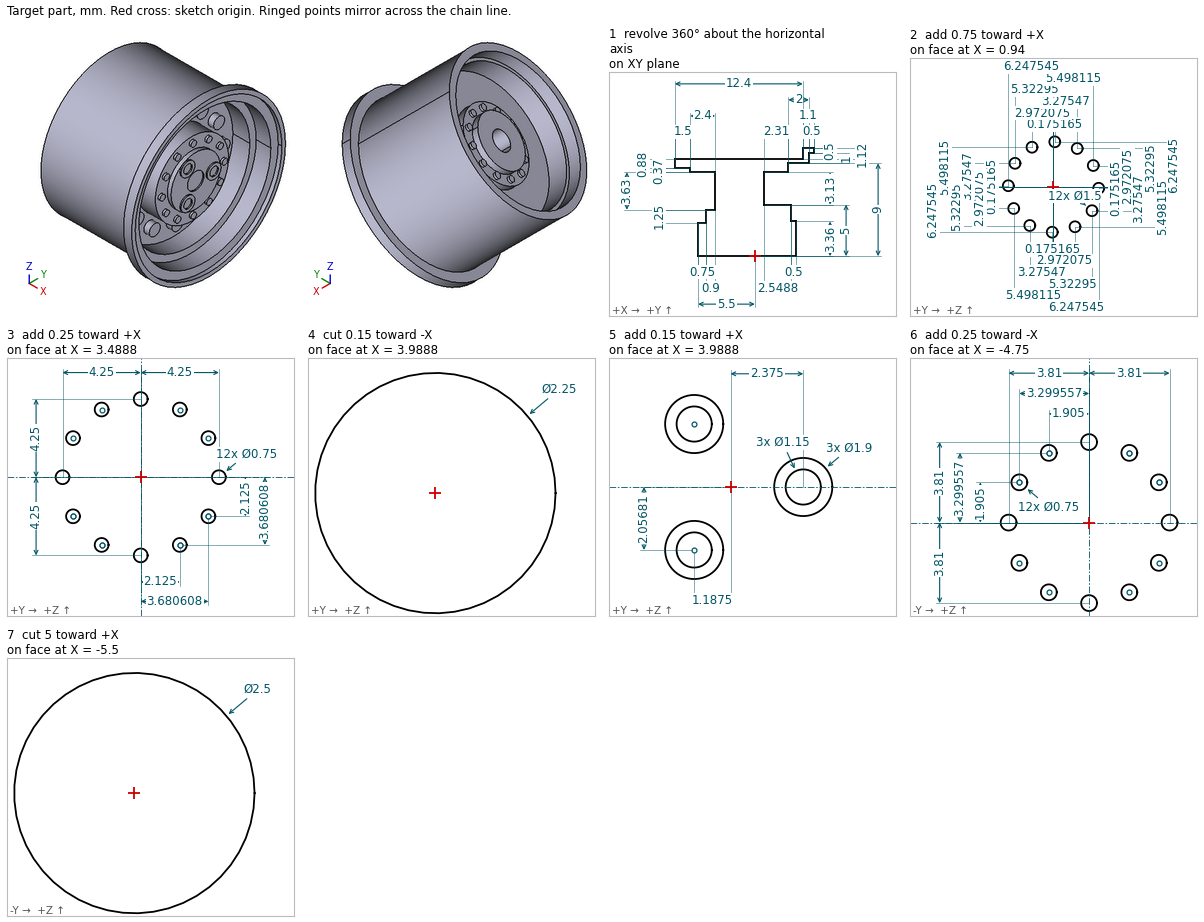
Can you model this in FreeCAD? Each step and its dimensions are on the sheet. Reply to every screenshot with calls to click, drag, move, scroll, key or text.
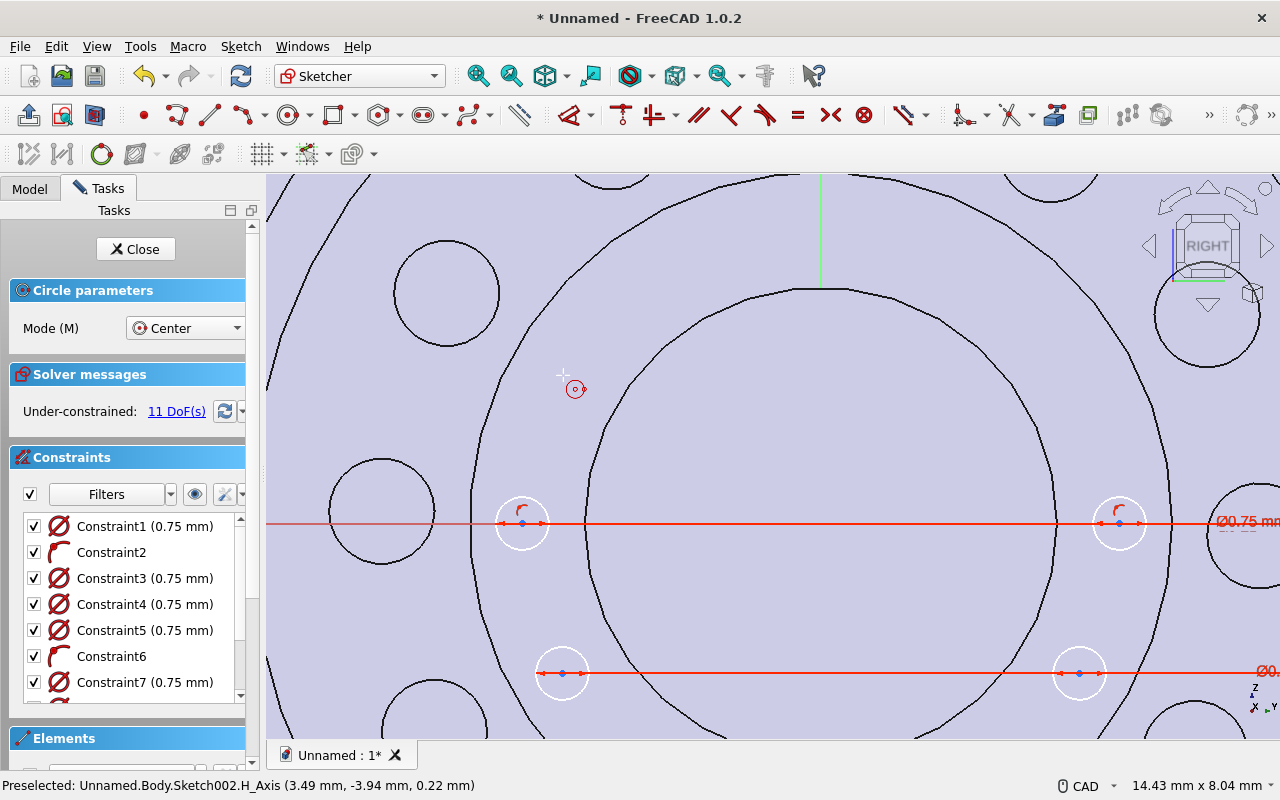
click(562, 374)
move(581, 356)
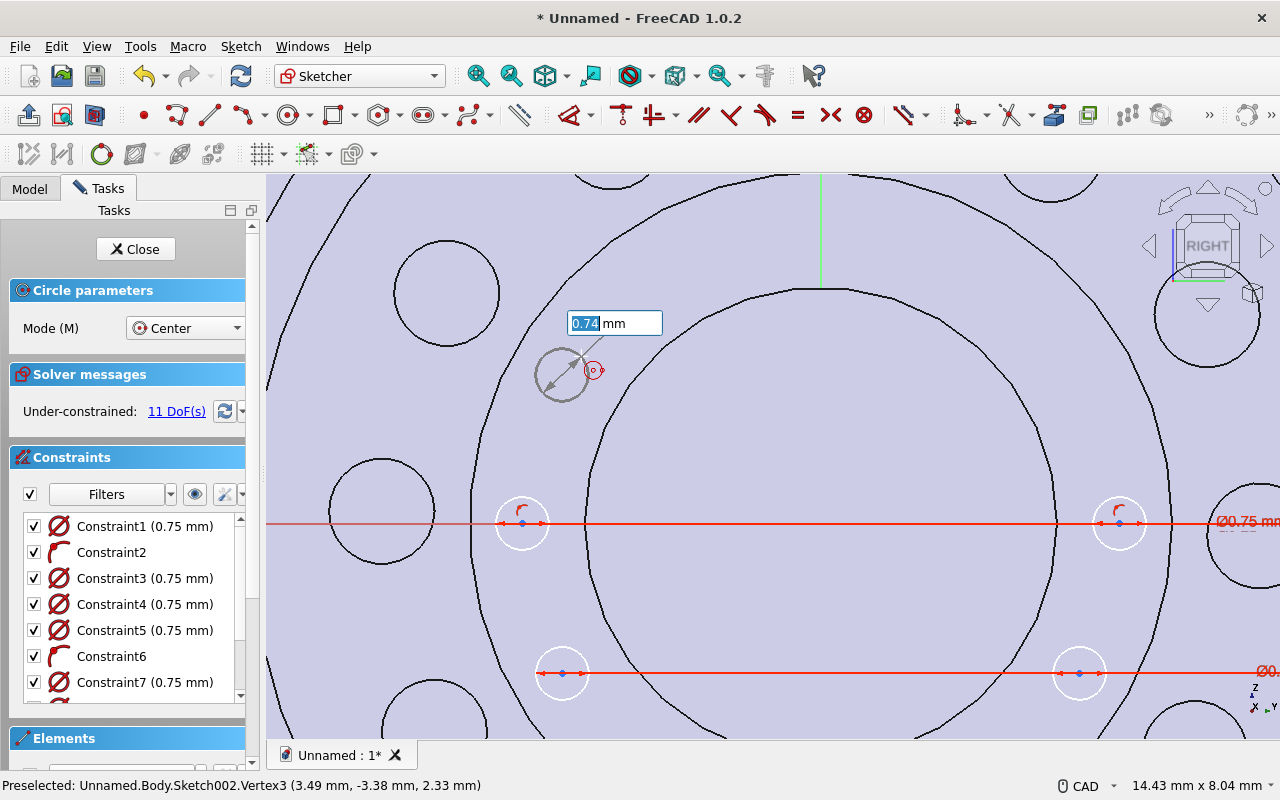
text(0.75)
key(Return)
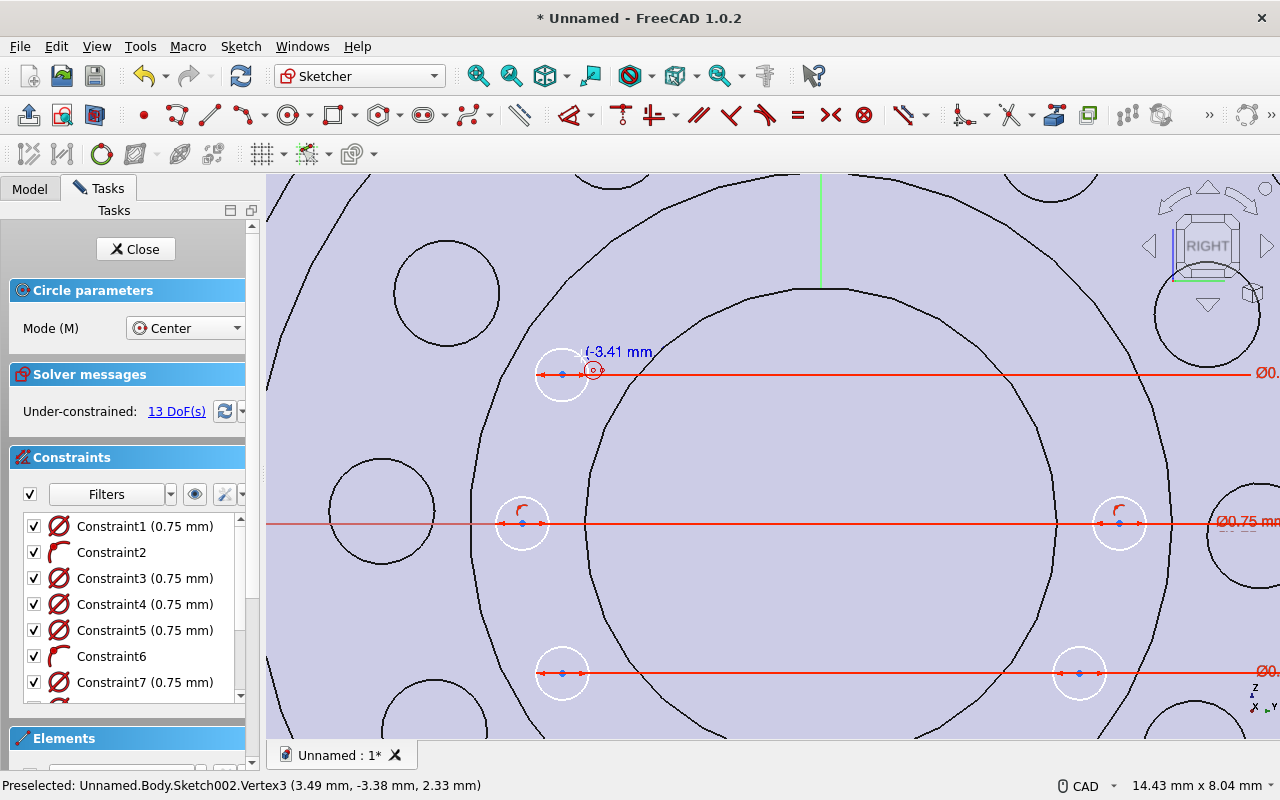
click(671, 265)
move(690, 246)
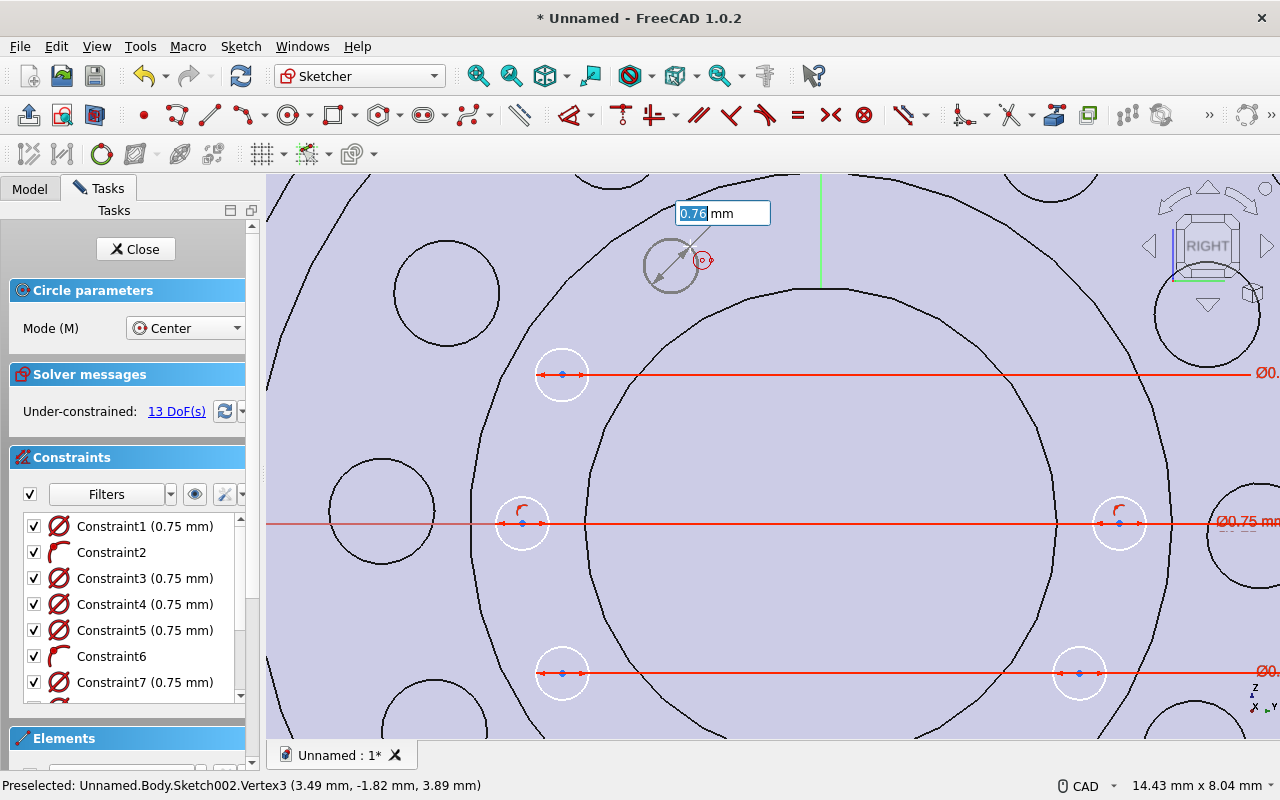
text(0.75)
key(Return)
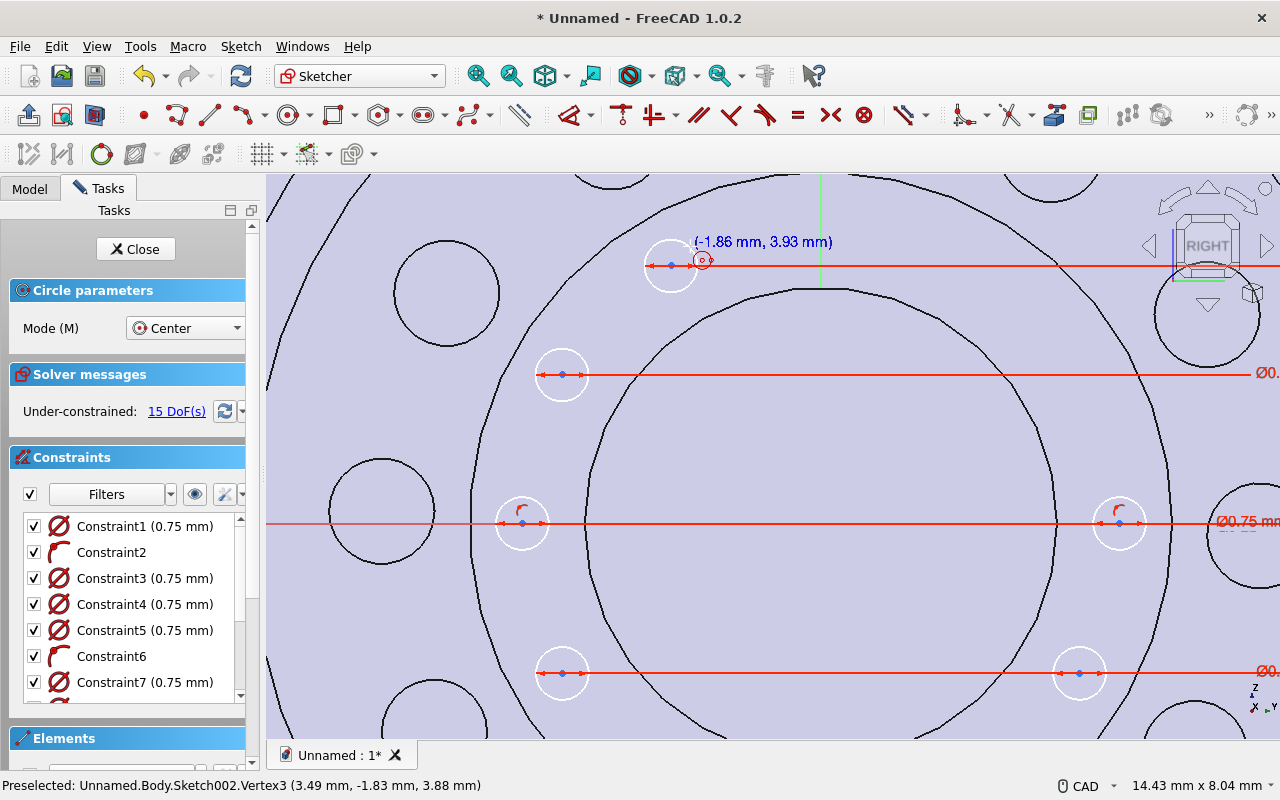
click(821, 225)
move(839, 206)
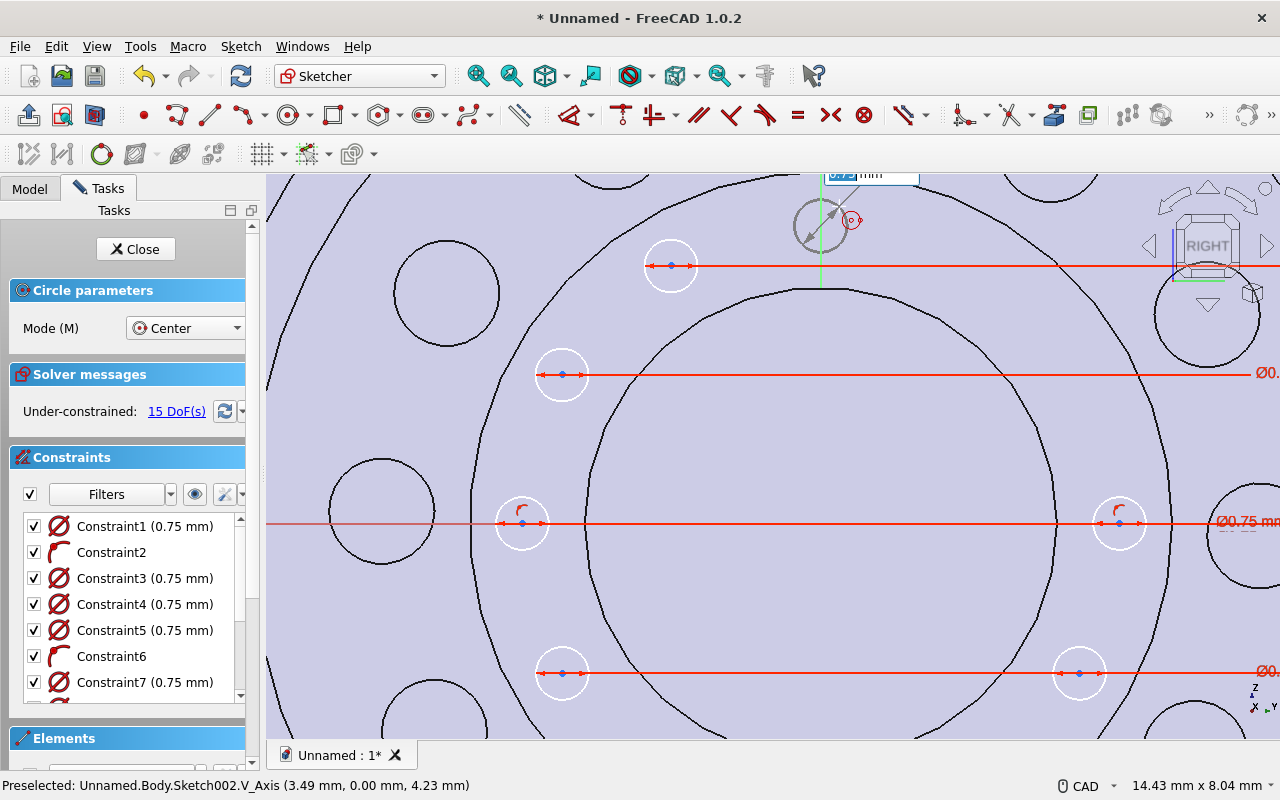
text(0.75)
key(Return)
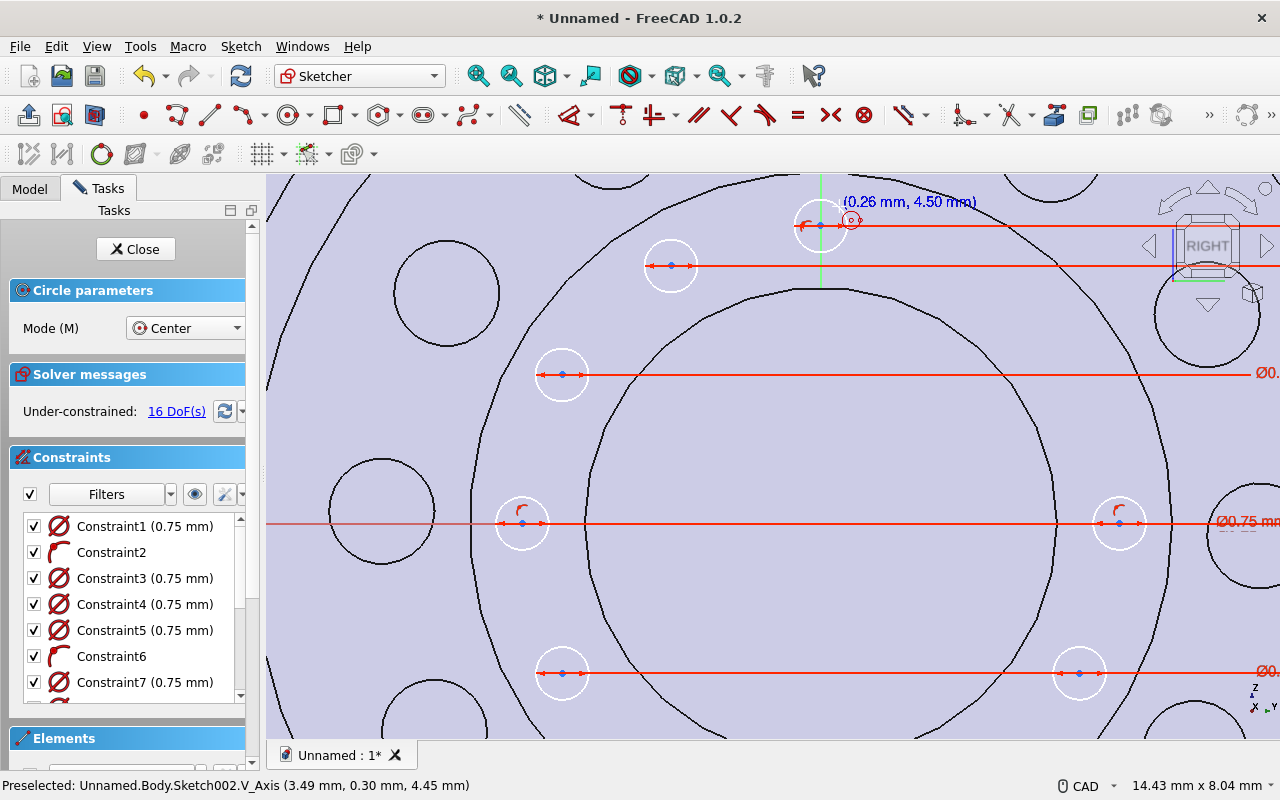
click(970, 265)
move(989, 246)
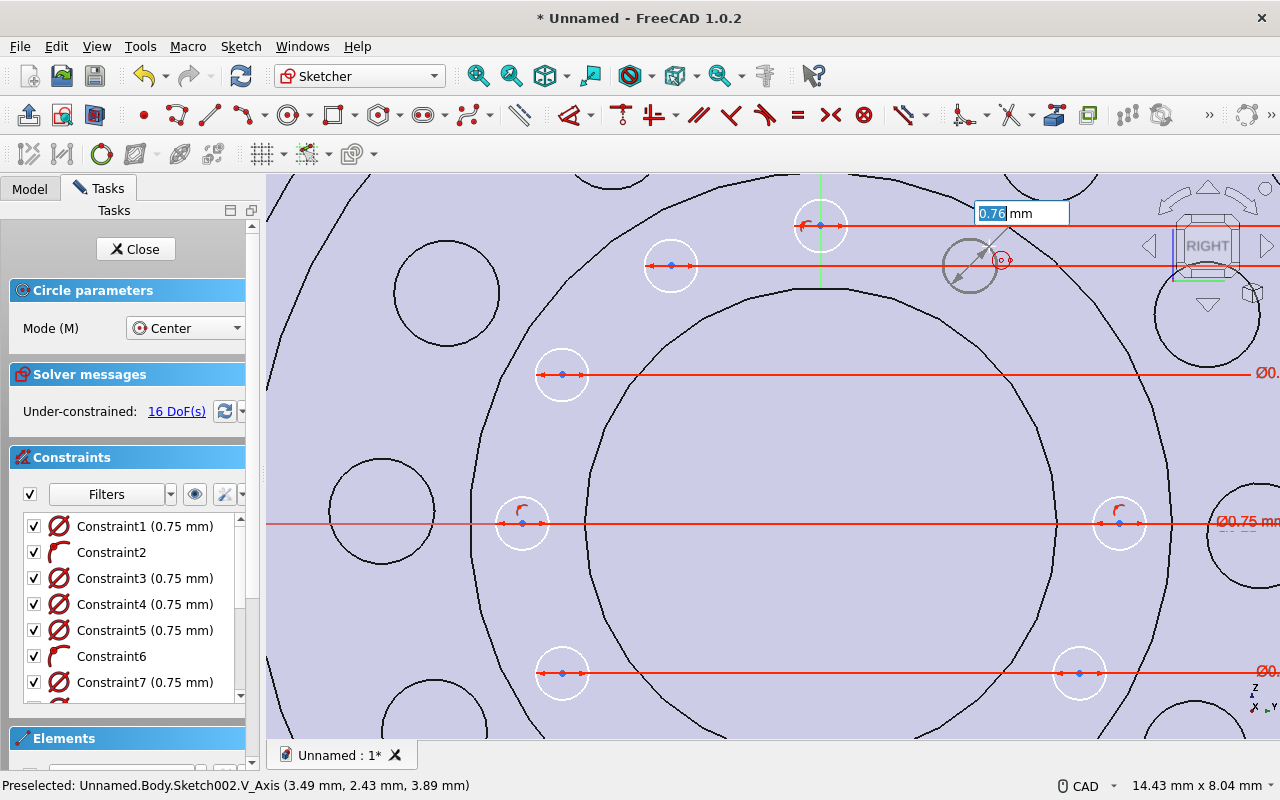
text(0.75)
key(Return)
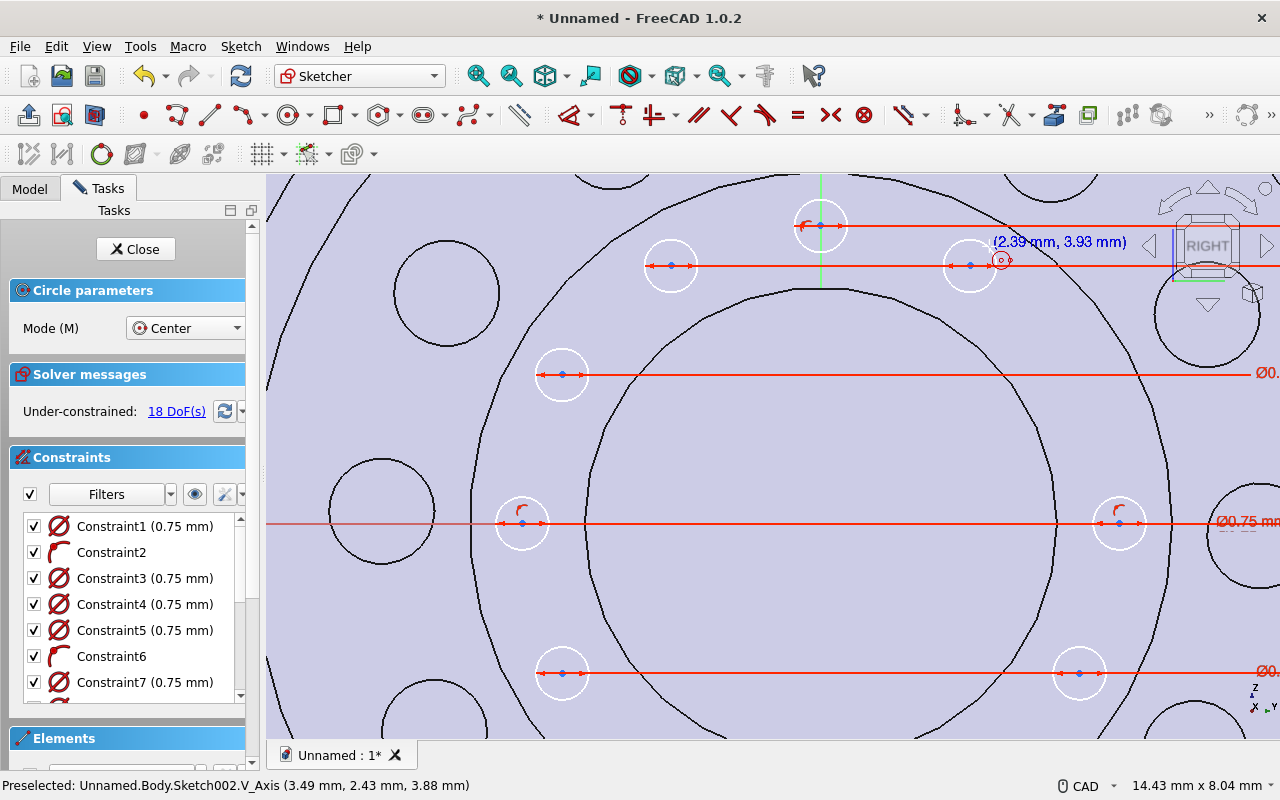
click(1079, 374)
move(1098, 356)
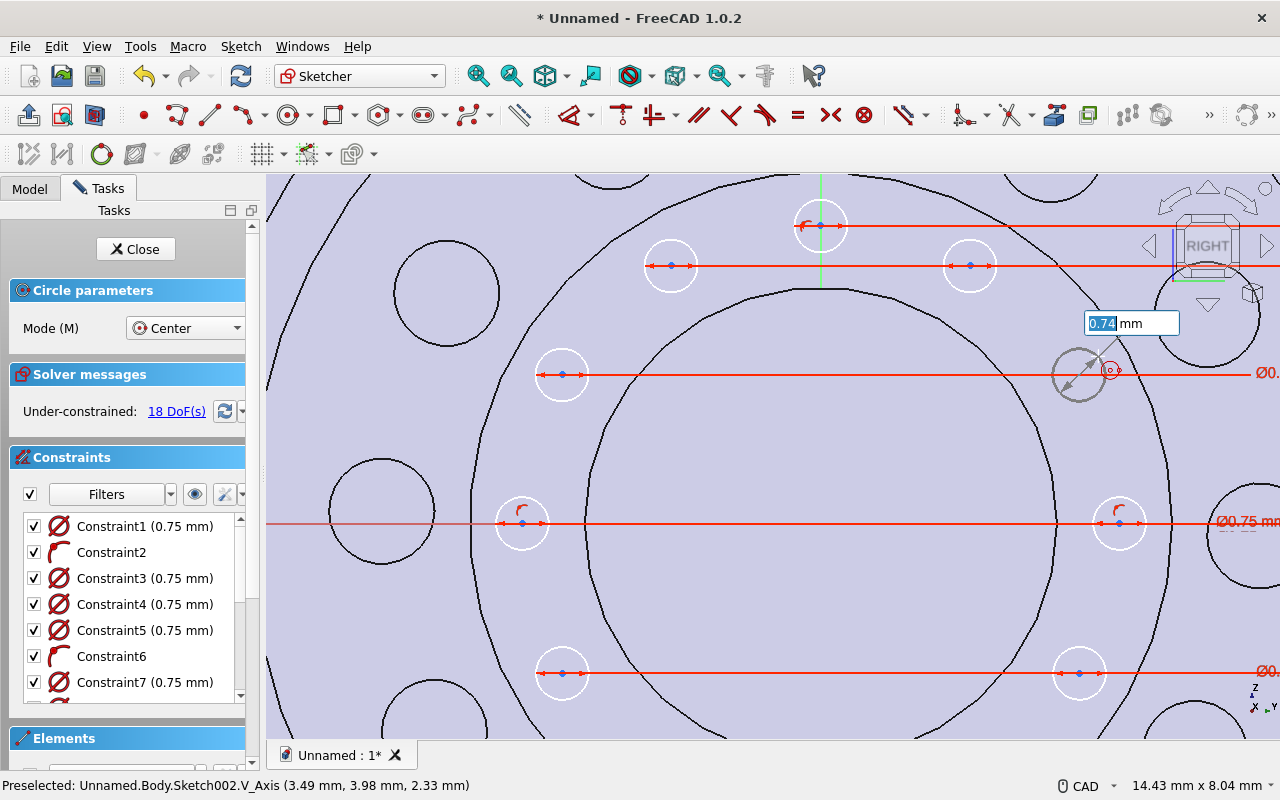
text(0.75)
key(Return)
key(Escape)